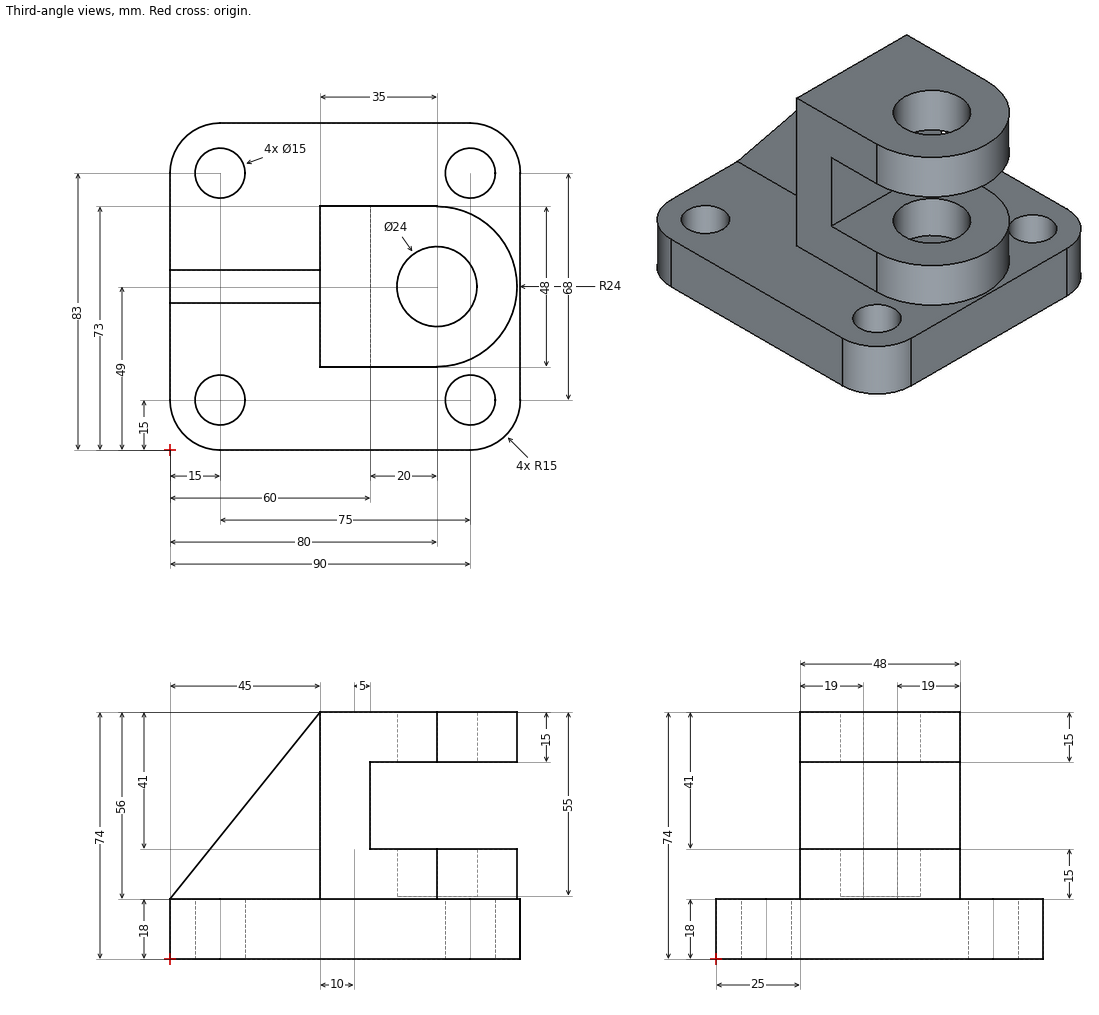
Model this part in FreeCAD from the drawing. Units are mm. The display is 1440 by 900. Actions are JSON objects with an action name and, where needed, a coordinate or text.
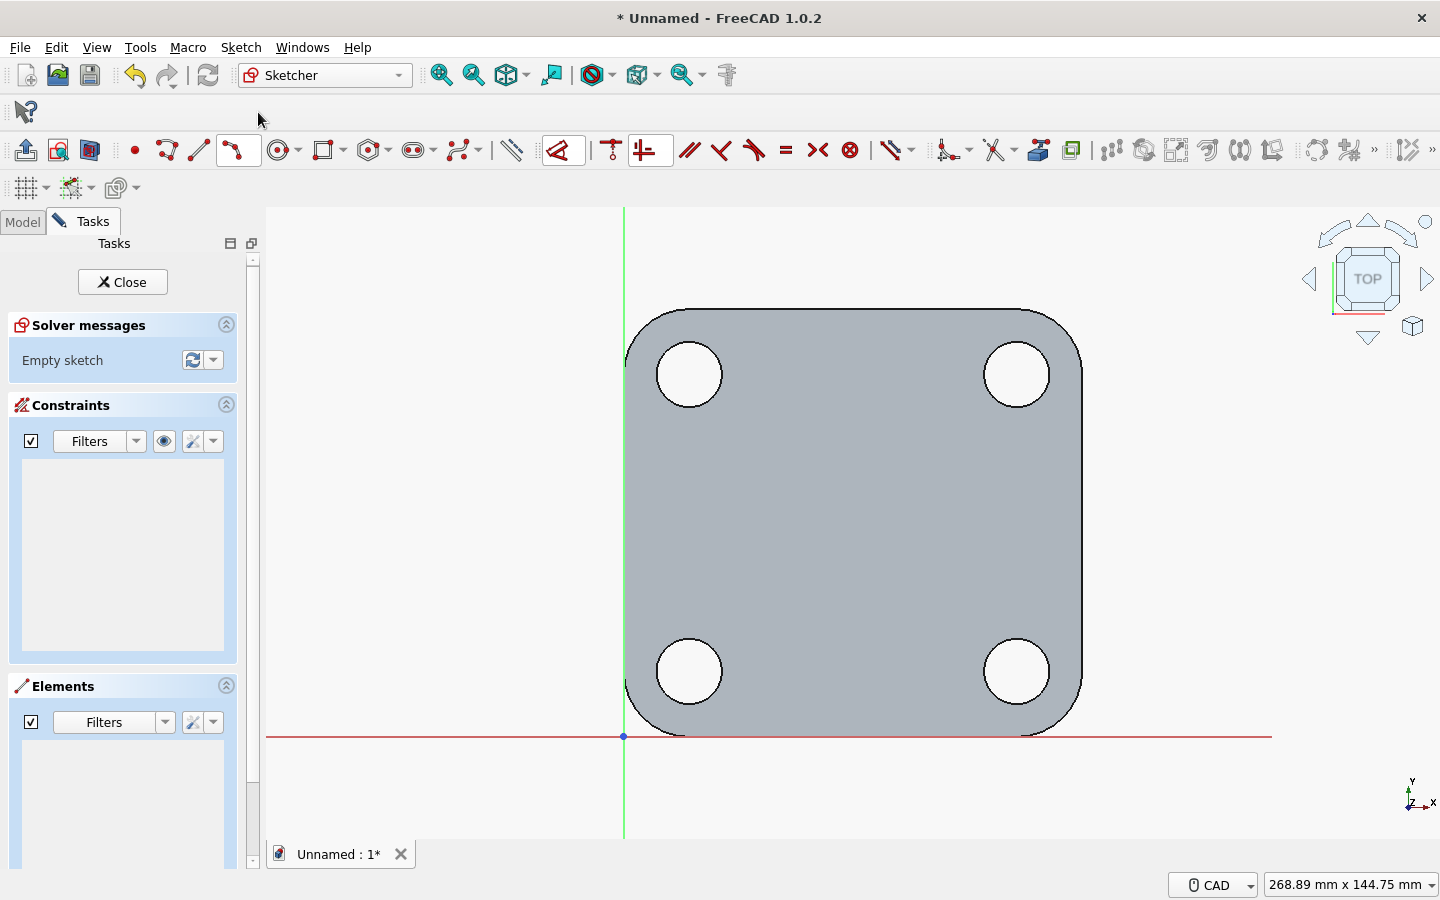
{"action": "left_click", "coordinate": [168, 150]}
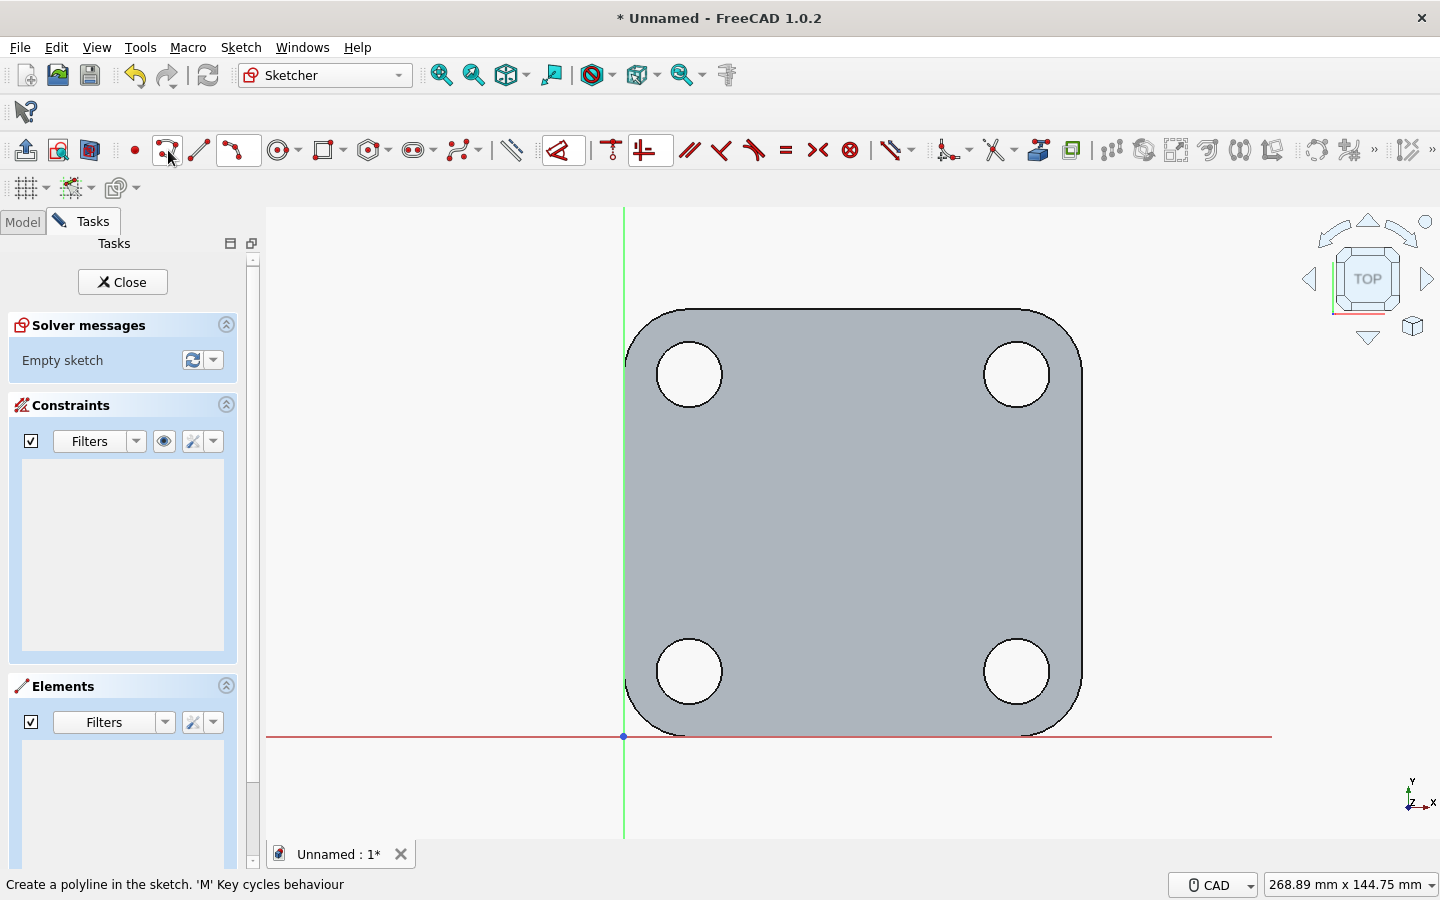
{"action": "left_click", "coordinate": [973, 418]}
{"action": "left_click", "coordinate": [820, 418]}
{"action": "left_click", "coordinate": [820, 628]}
{"action": "left_click", "coordinate": [973, 628]}
{"action": "right_click", "coordinate": [973, 628]}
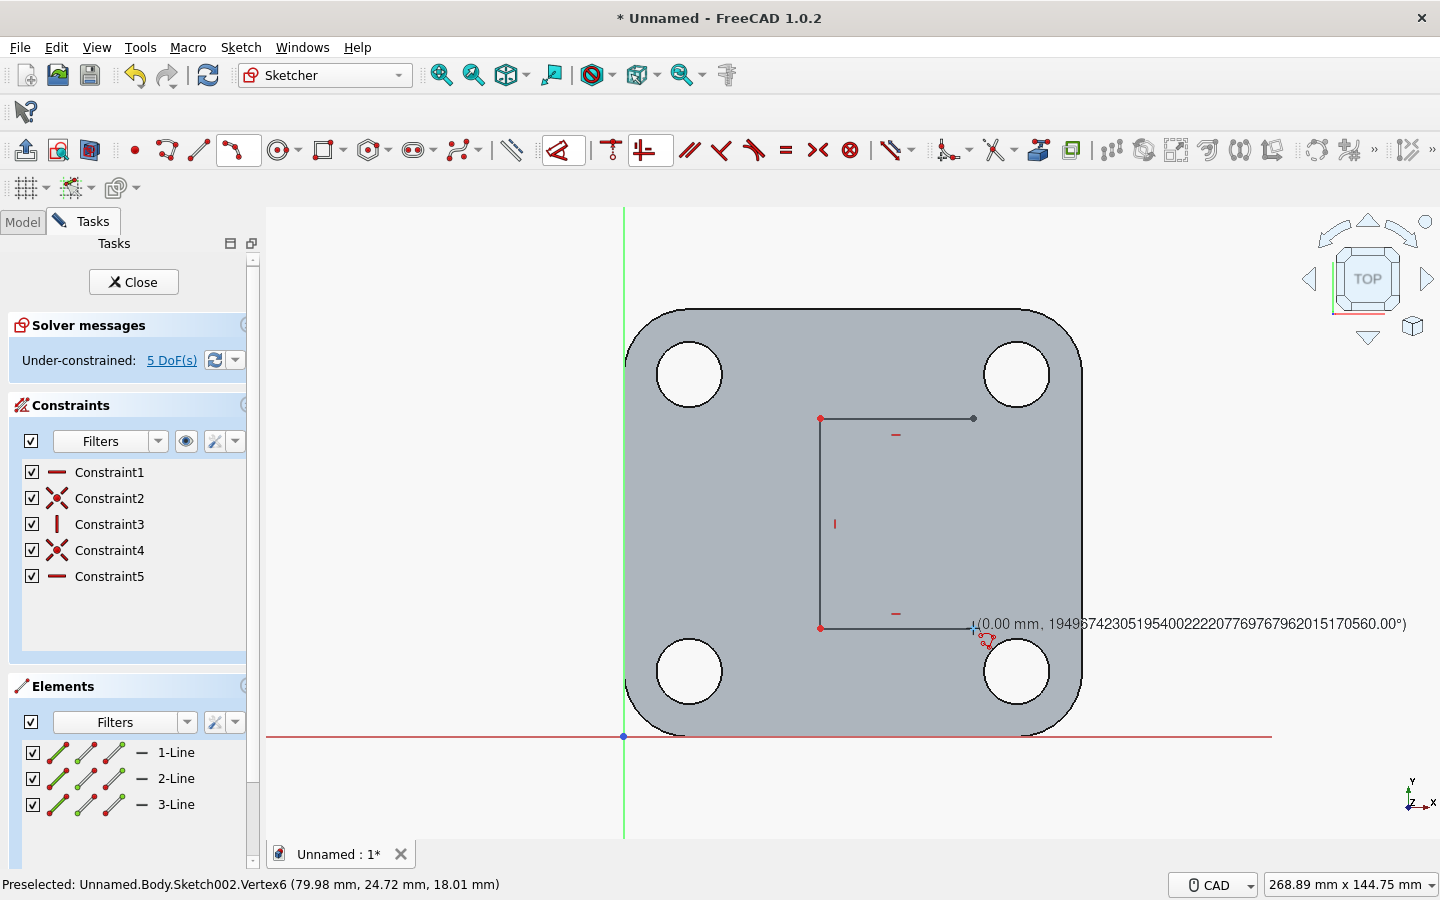
{"action": "left_click", "coordinate": [232, 150]}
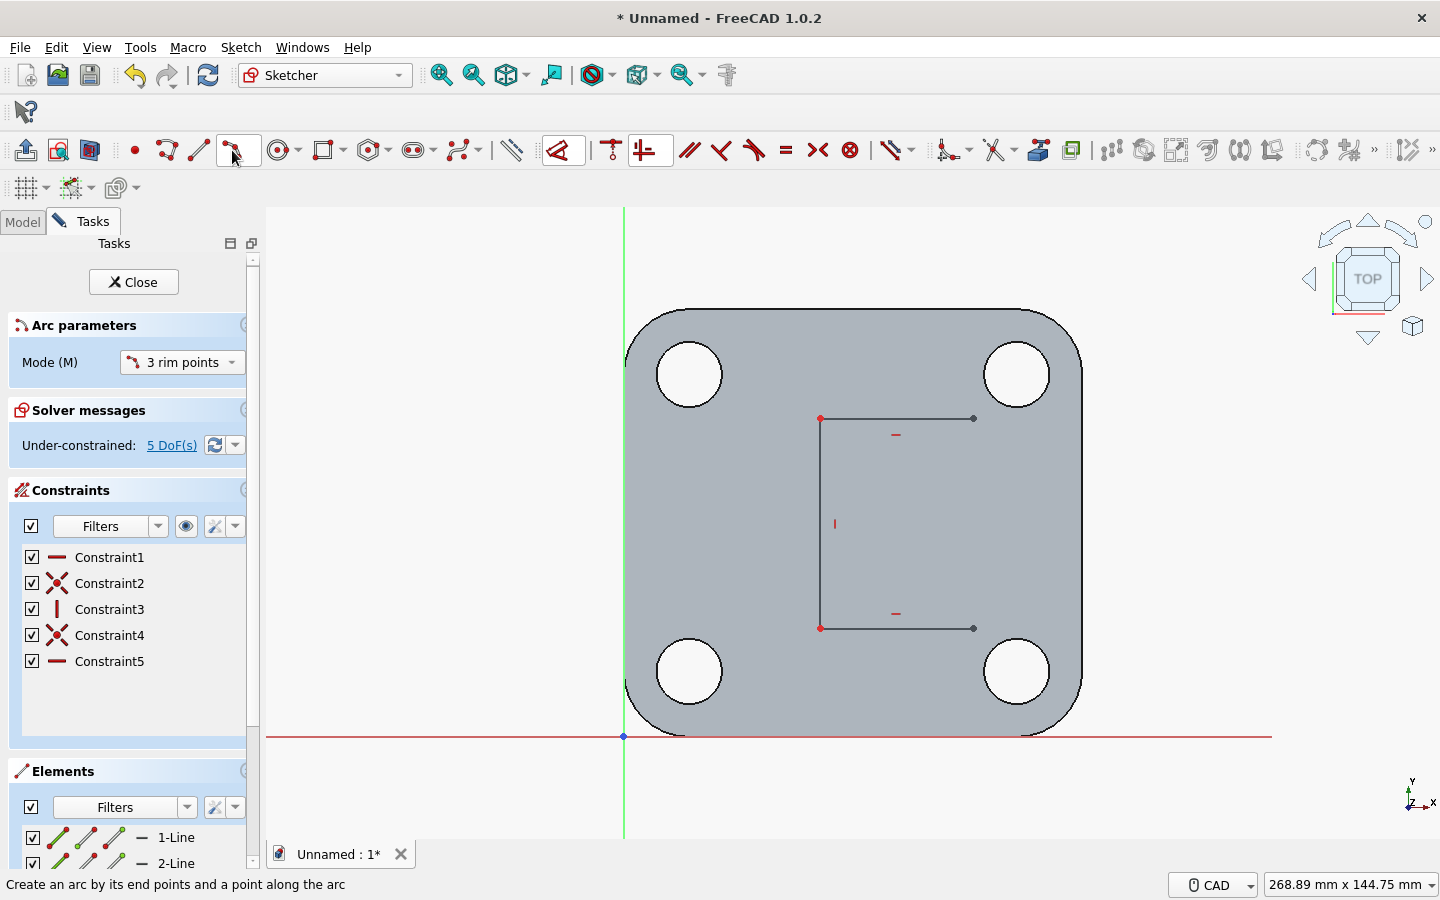
{"action": "left_click", "coordinate": [973, 629]}
{"action": "left_click", "coordinate": [973, 419]}
{"action": "left_click", "coordinate": [1078, 523]}
{"action": "key", "text": "Escape"}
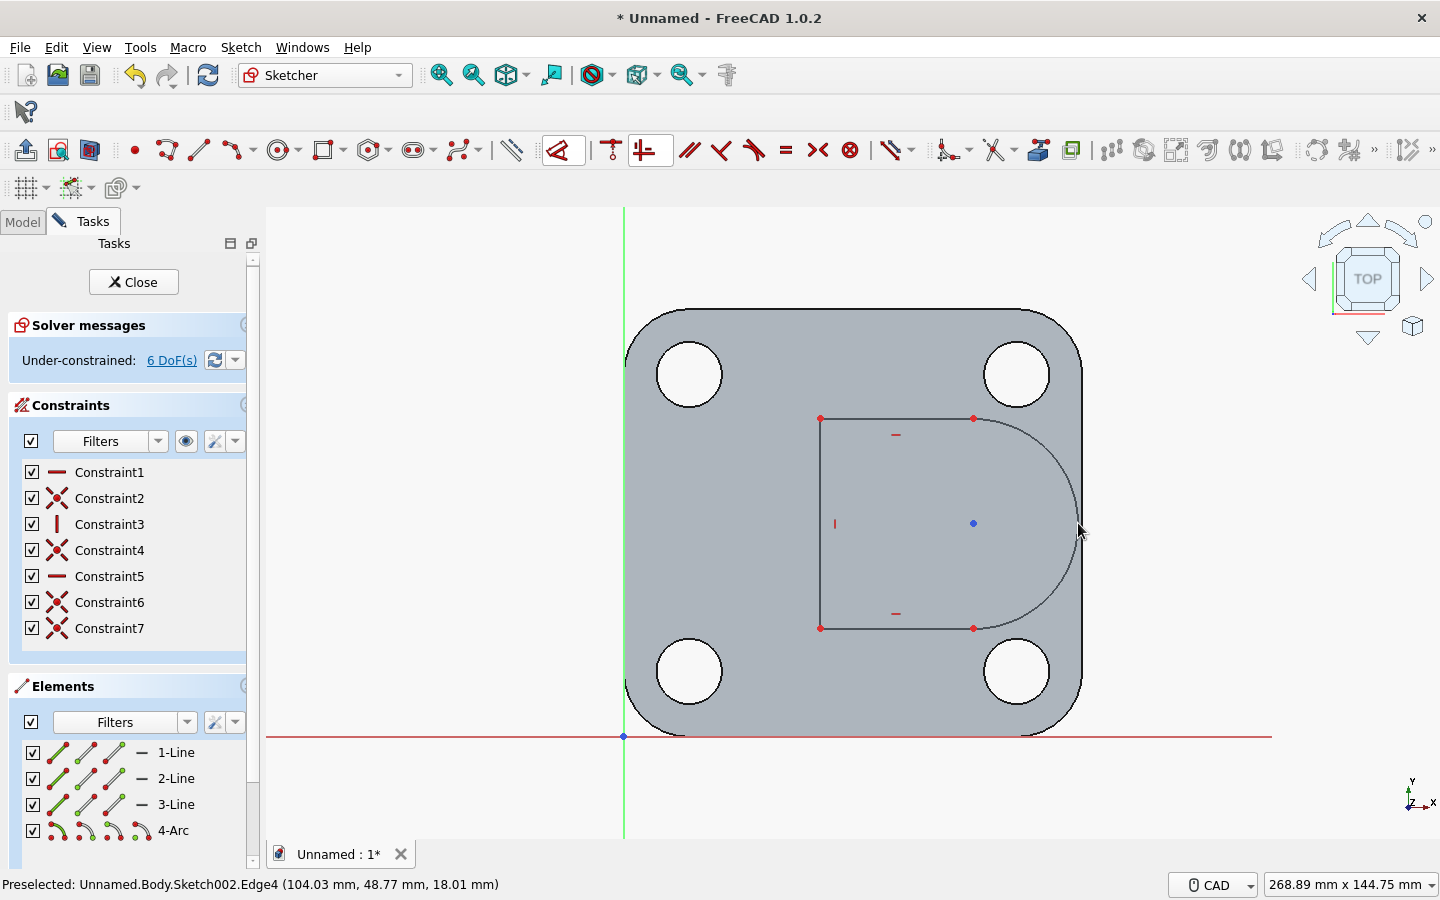
{"action": "left_click", "coordinate": [927, 419]}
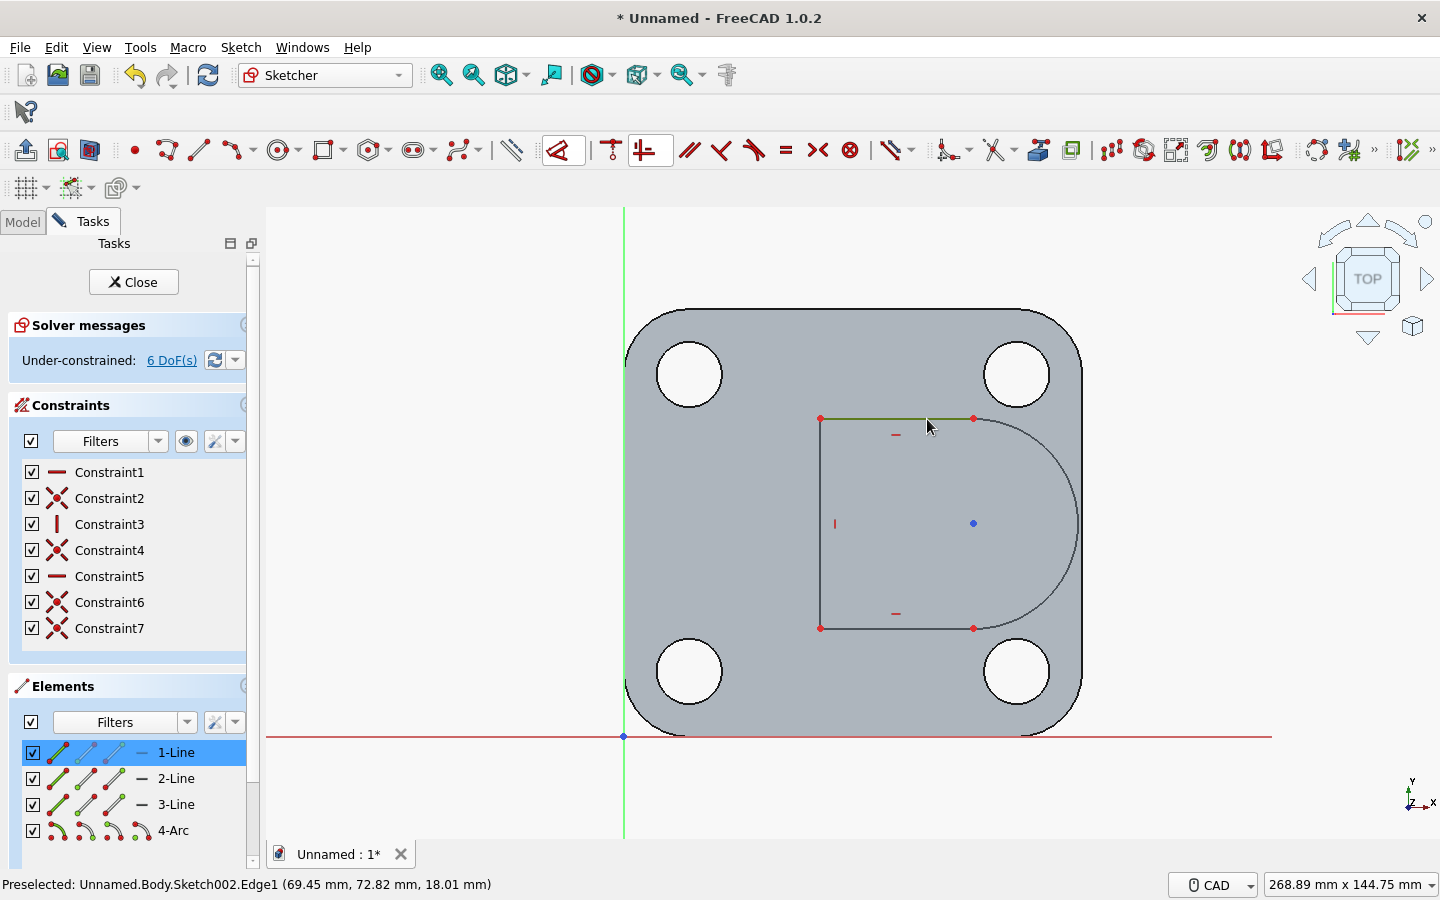
{"action": "left_click", "coordinate": [1058, 586]}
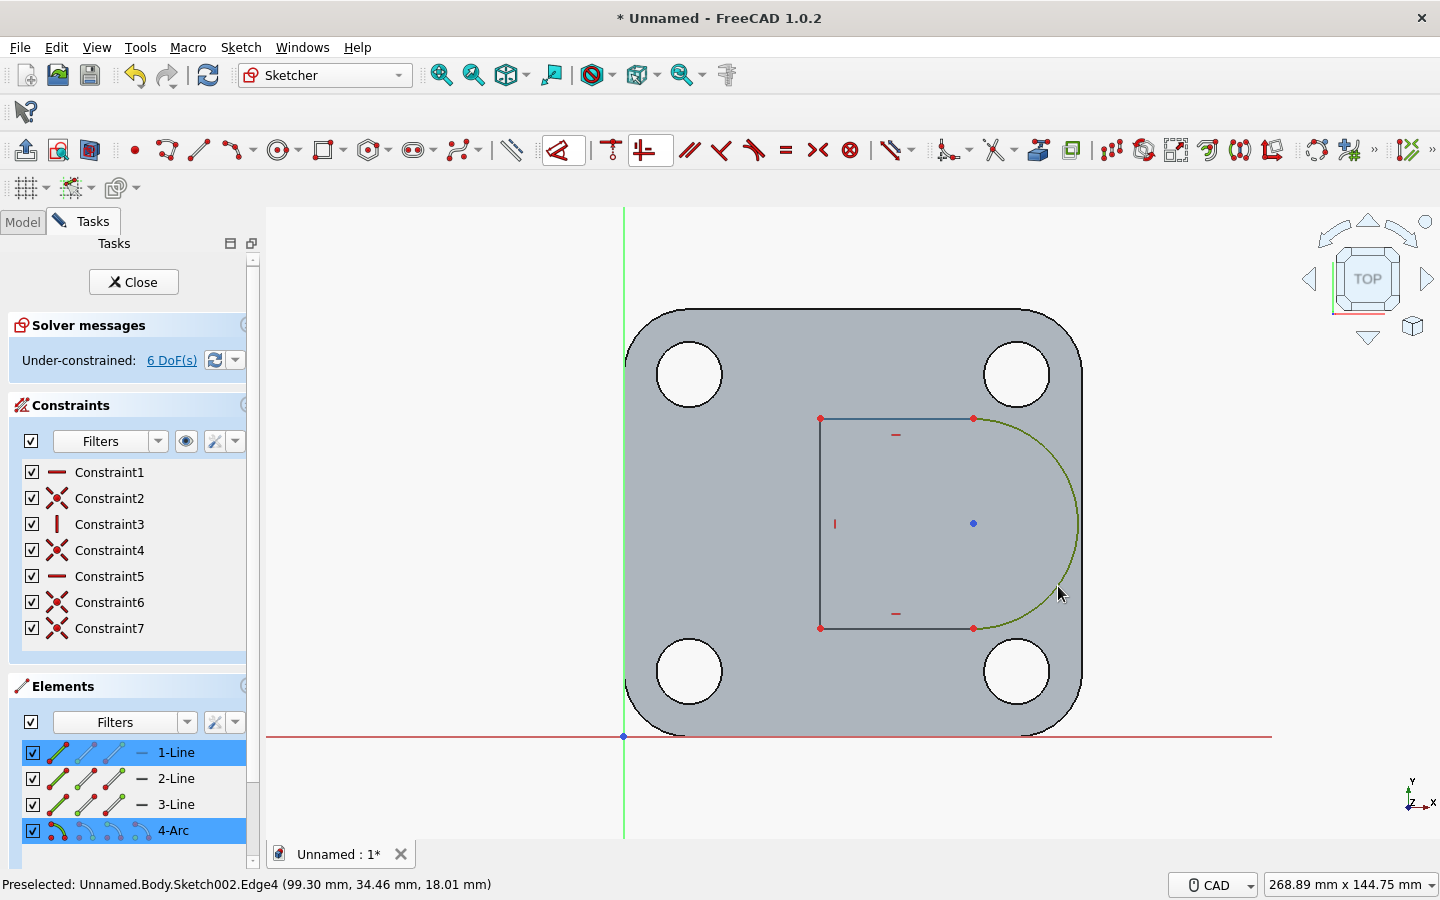
{"action": "left_click", "coordinate": [754, 150]}